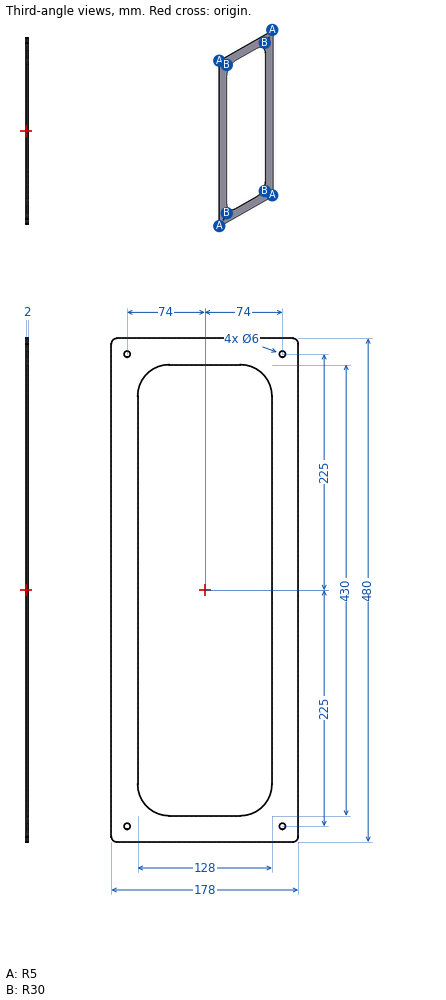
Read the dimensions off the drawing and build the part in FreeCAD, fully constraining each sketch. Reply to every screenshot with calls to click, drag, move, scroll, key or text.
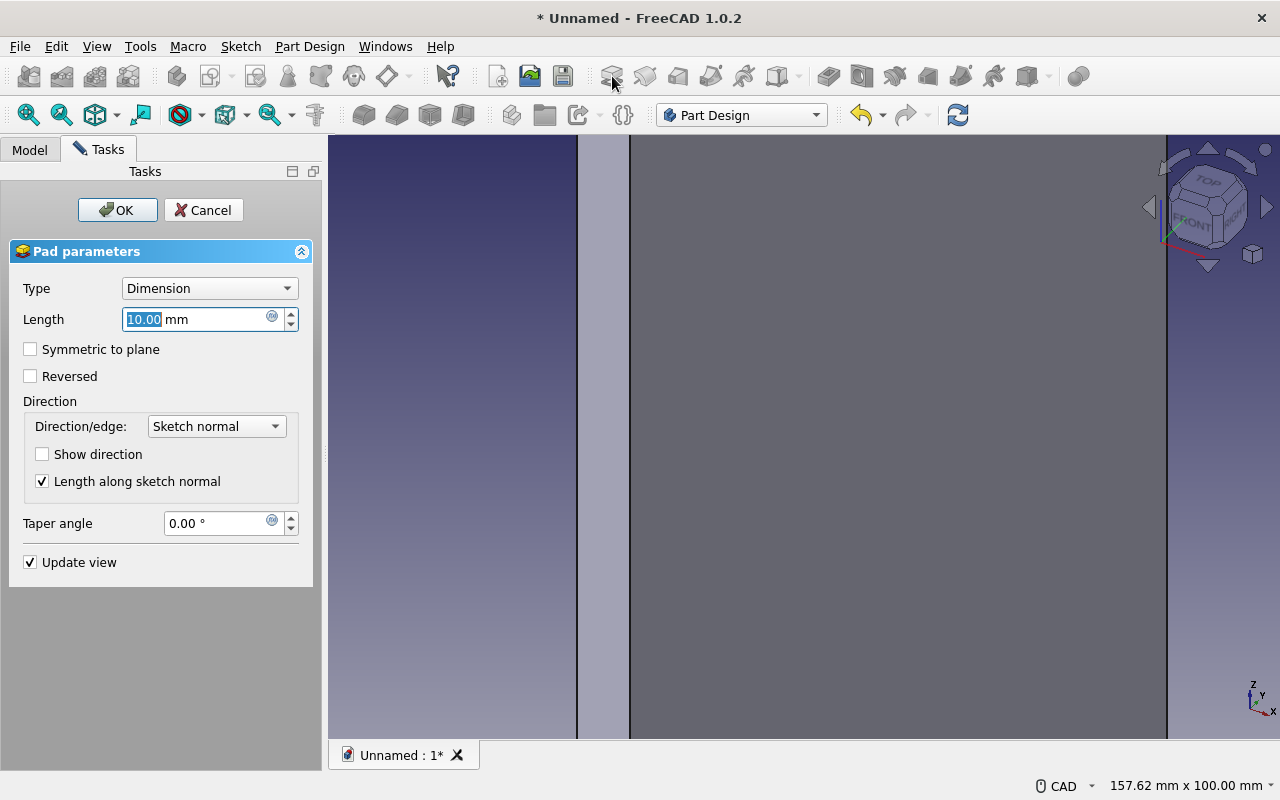
text(2)
key(Tab)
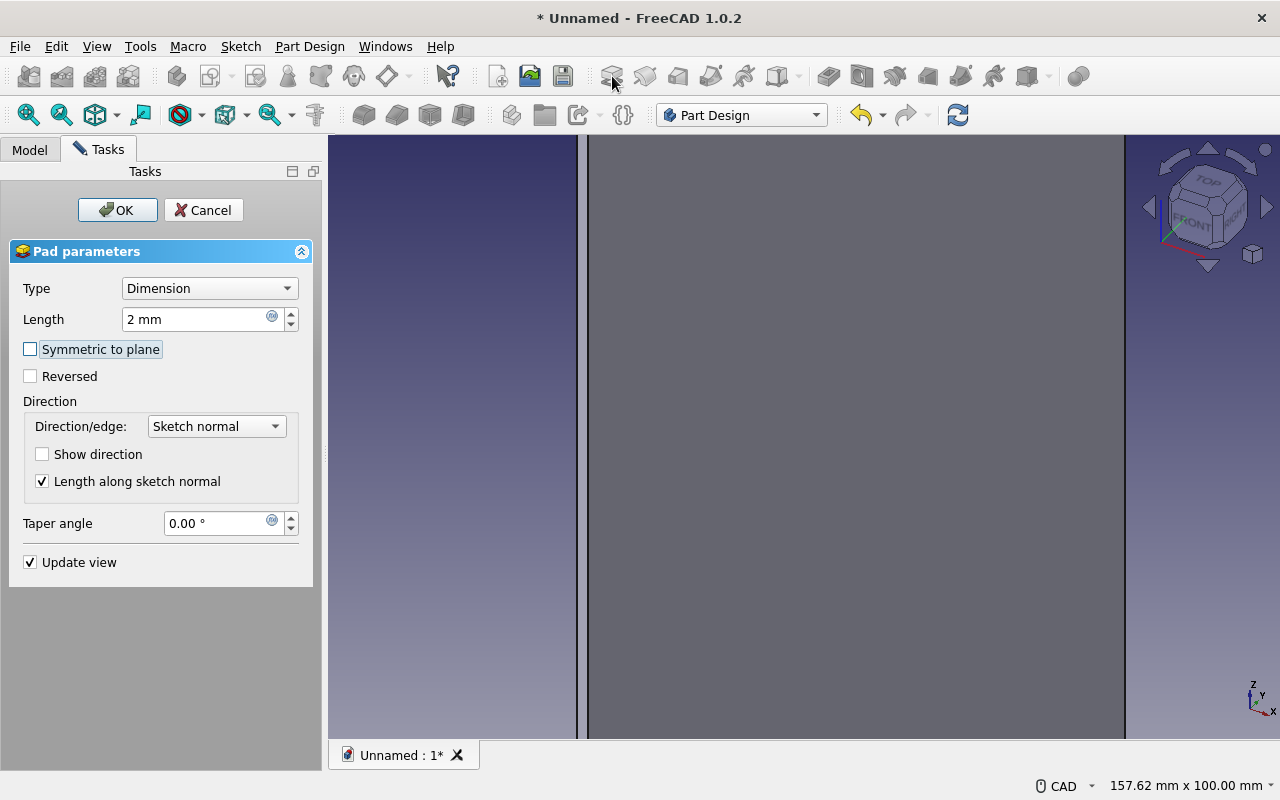
click(118, 210)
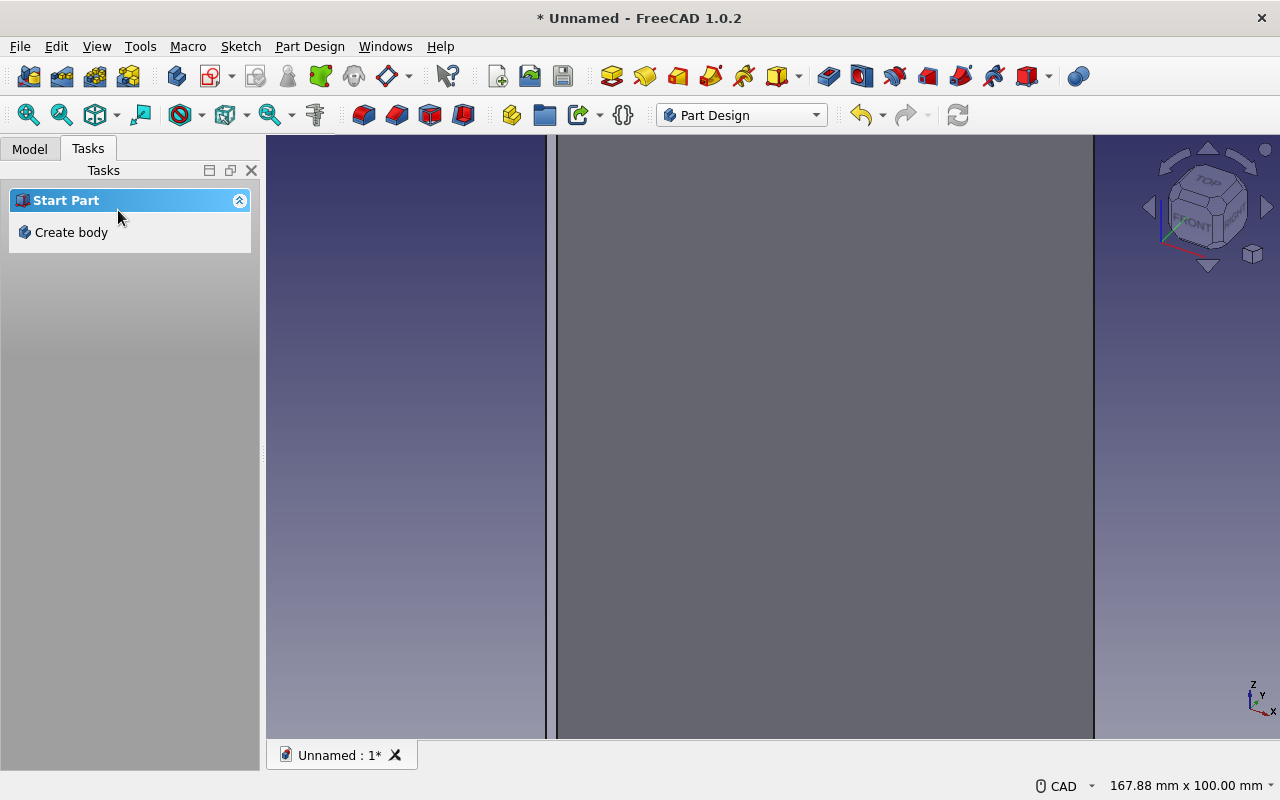
key(v)
key(f)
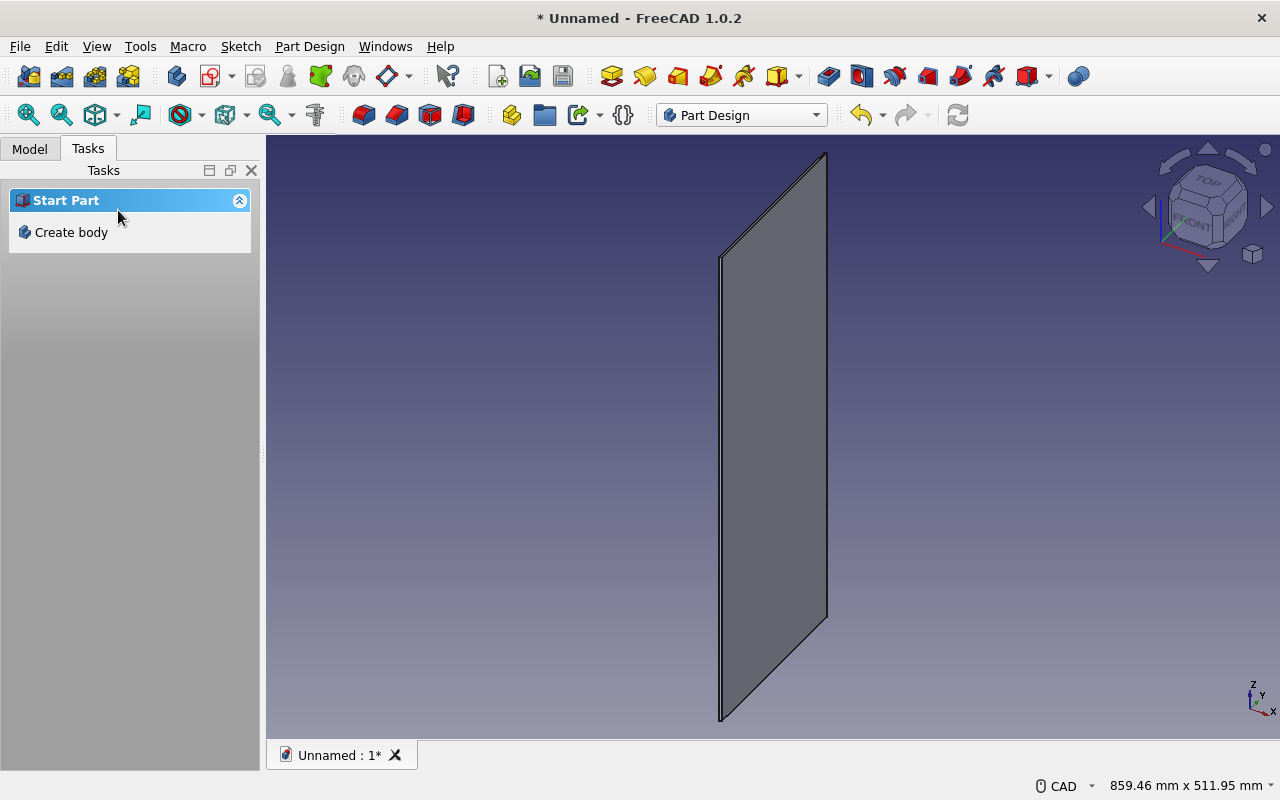
click(774, 569)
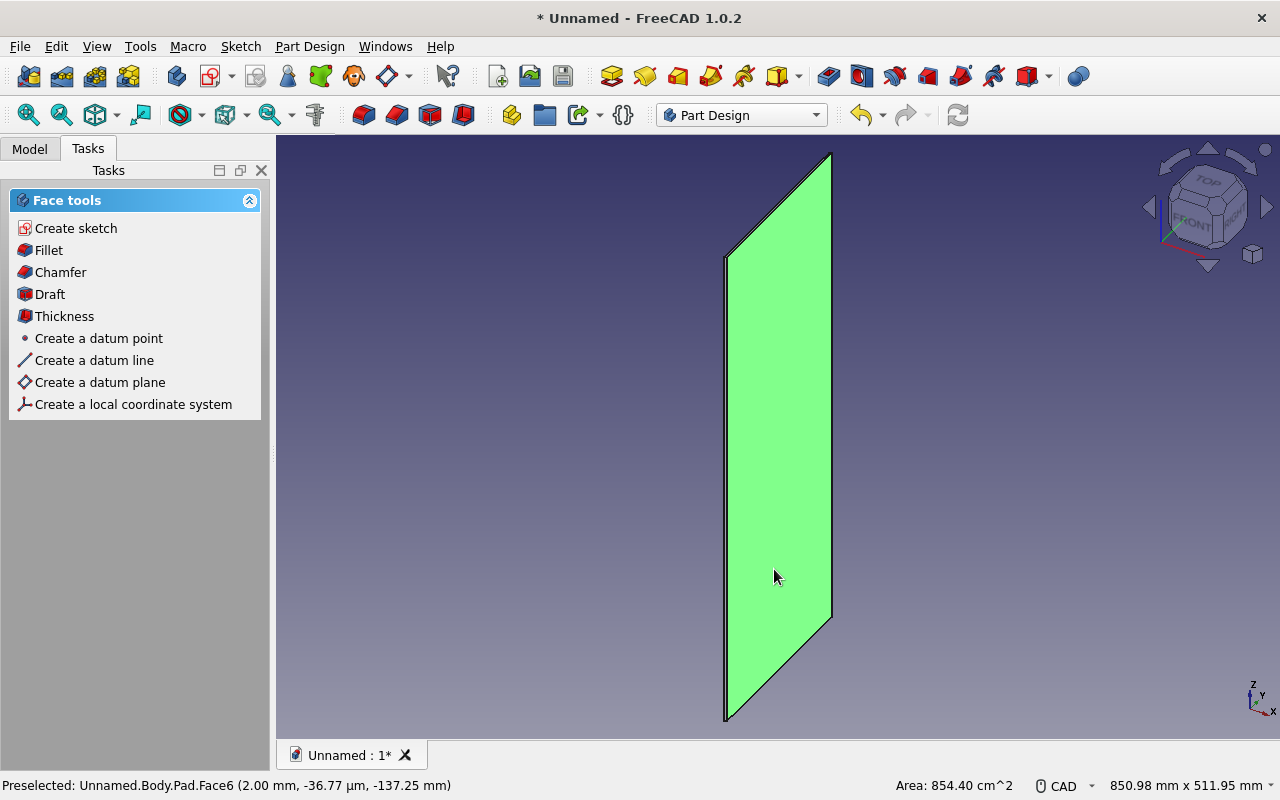
click(210, 76)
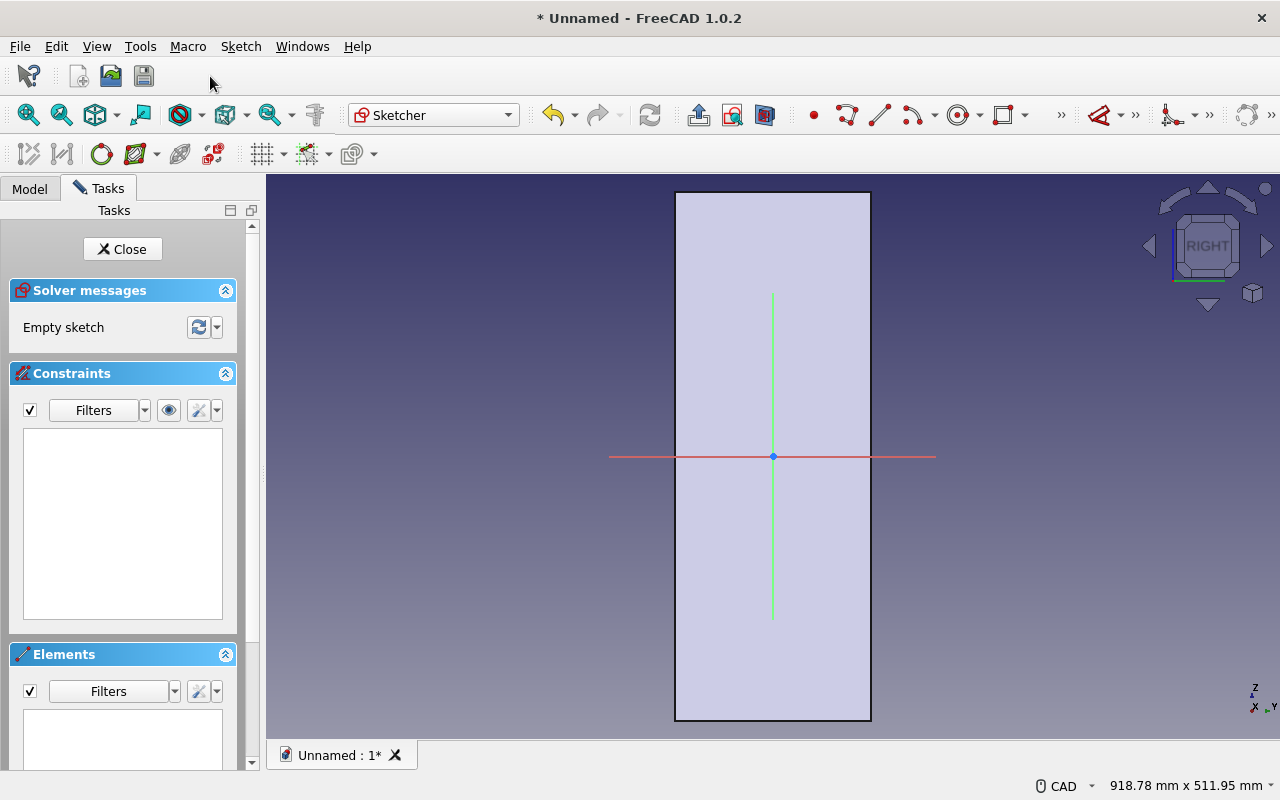
scroll(565, 457, down, 2)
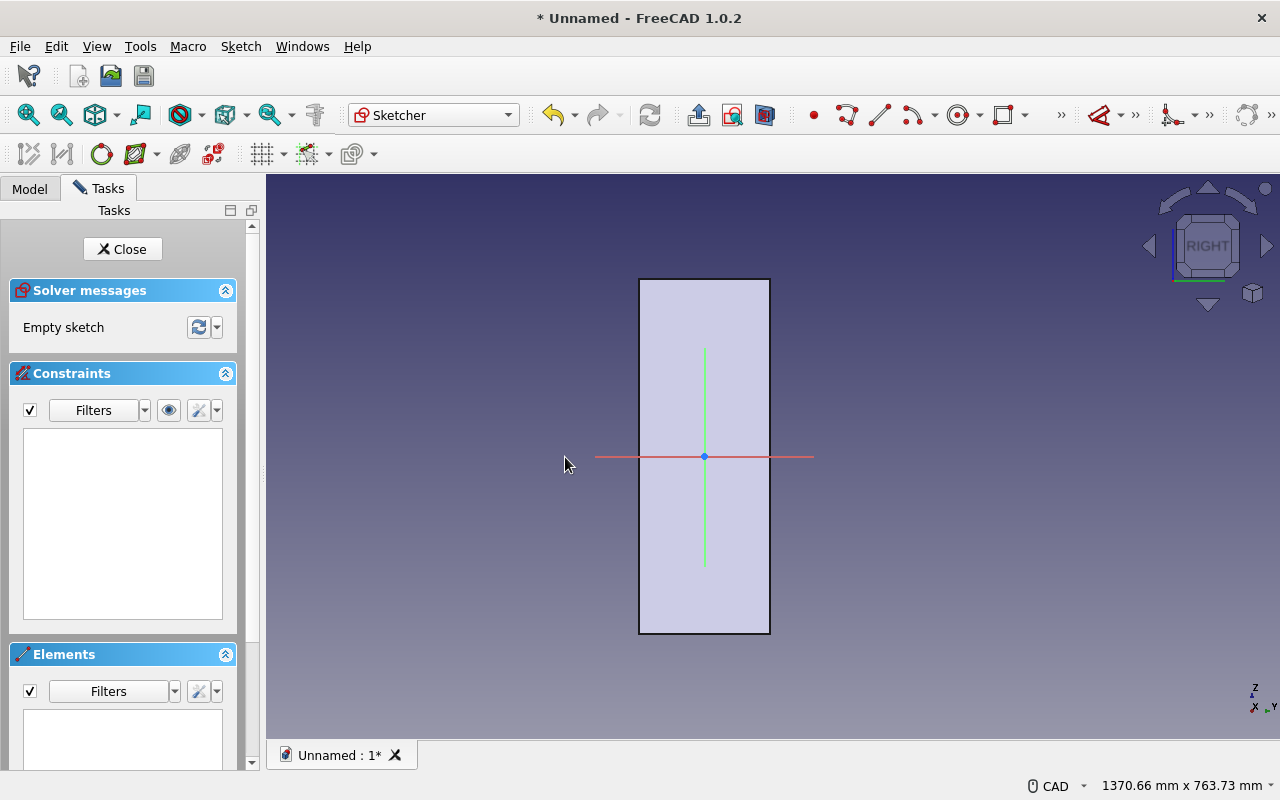
key(g)
key(c)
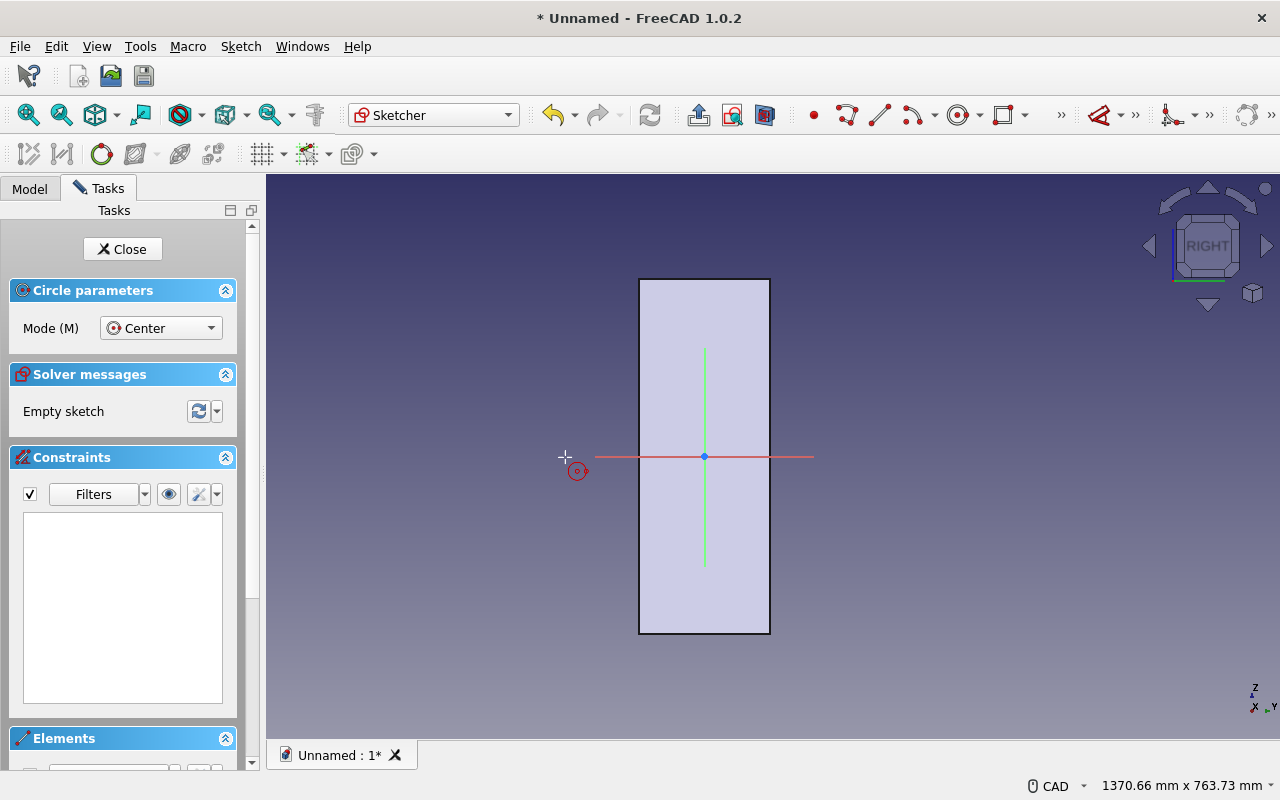
scroll(759, 290, up, 12)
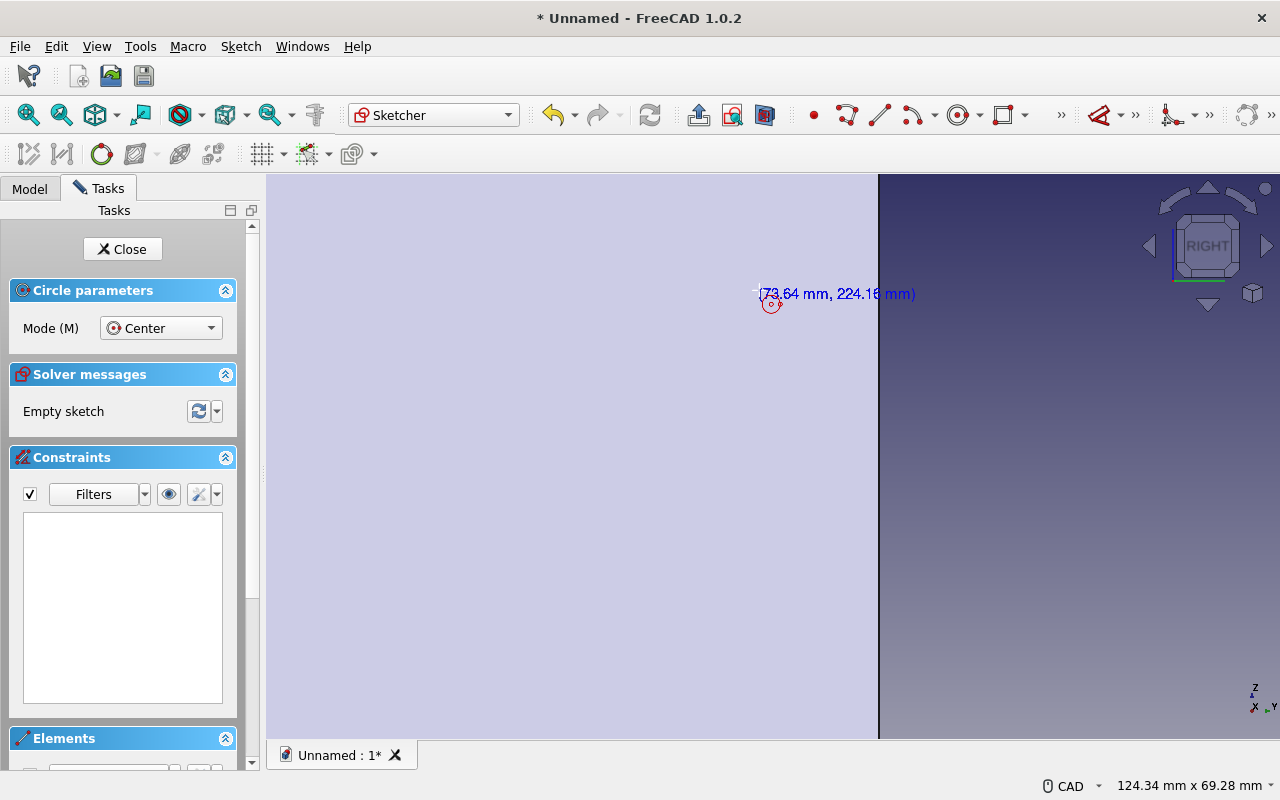
scroll(759, 290, down, 12)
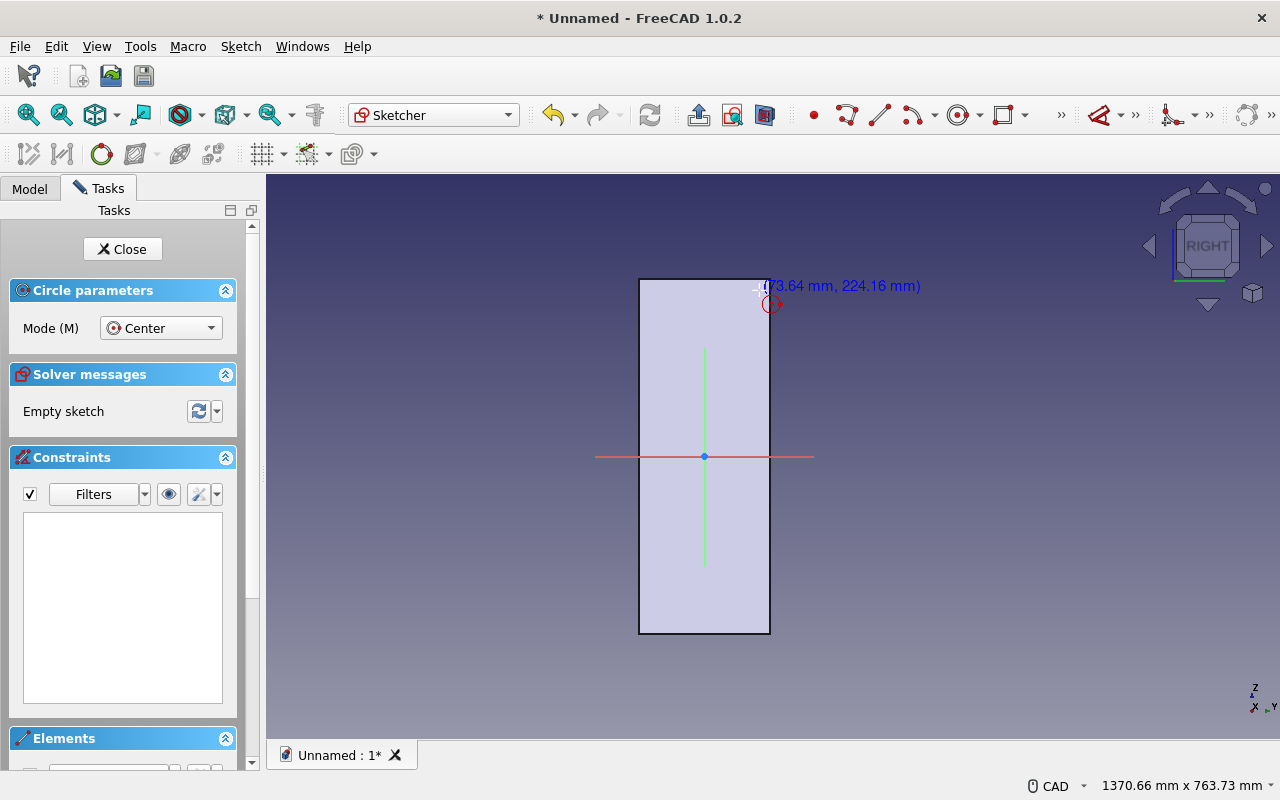
click(759, 290)
move(761, 289)